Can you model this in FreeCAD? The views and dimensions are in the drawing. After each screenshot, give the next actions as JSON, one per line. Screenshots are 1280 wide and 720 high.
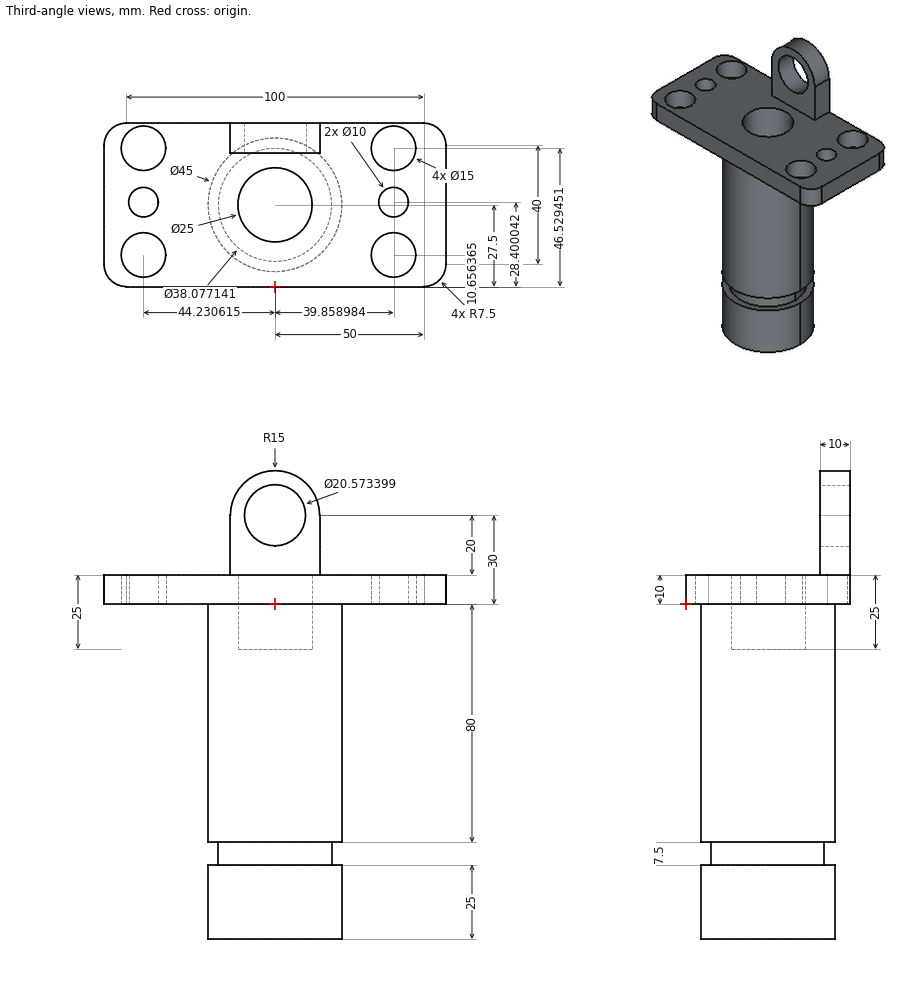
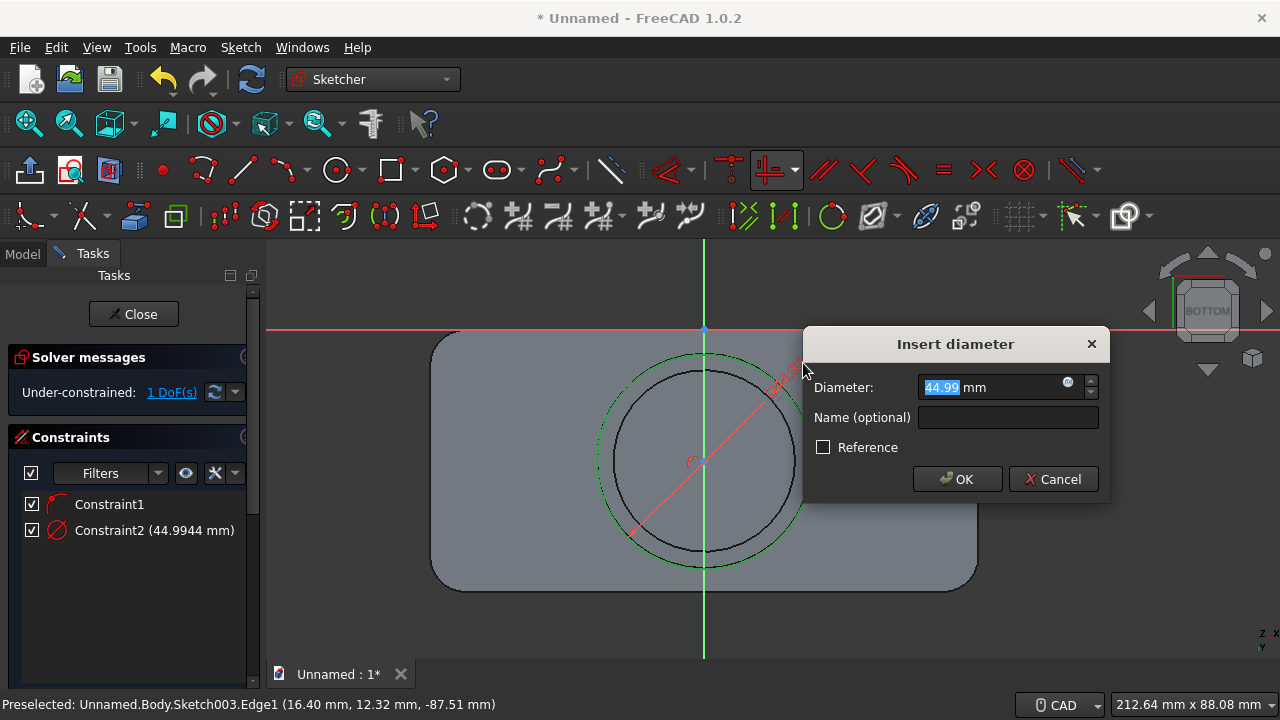
{"action": "type", "text": "45"}
{"action": "key", "text": "Return"}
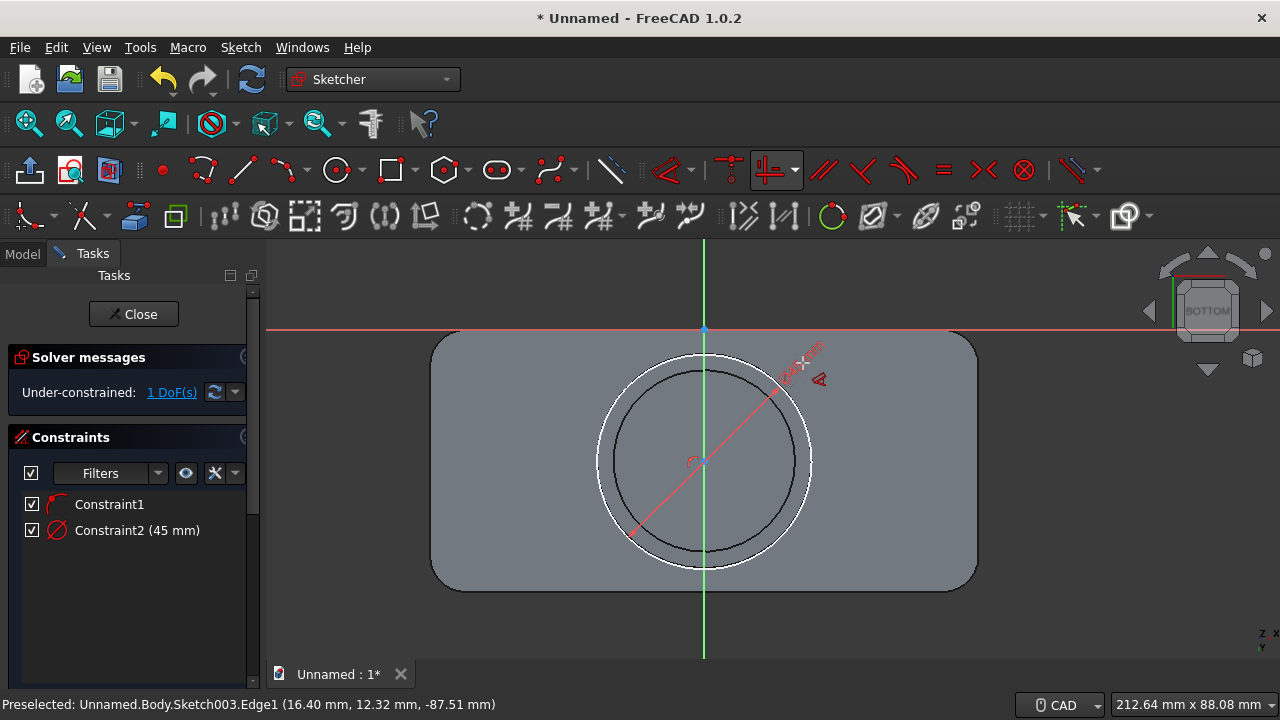
{"action": "left_click", "coordinate": [704, 462]}
{"action": "left_click", "coordinate": [738, 396]}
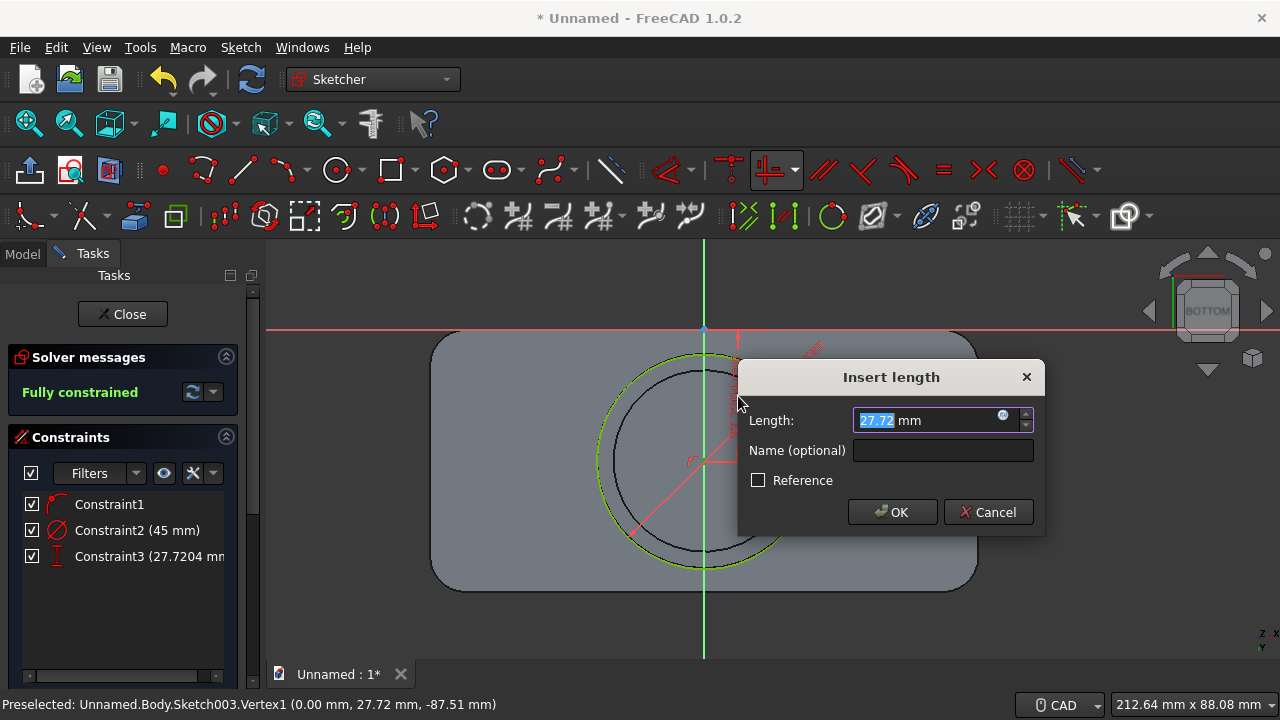
{"action": "type", "text": "27.5"}
{"action": "key", "text": "Return"}
{"action": "key", "text": "Escape"}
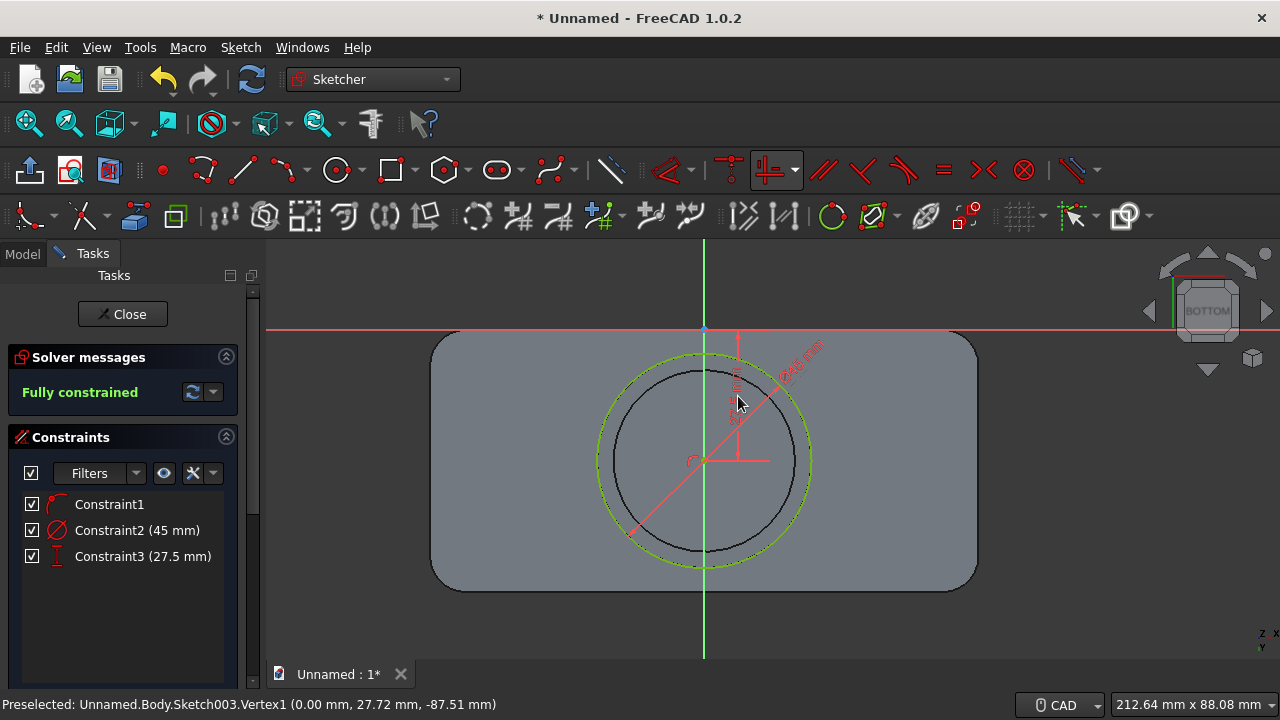
{"action": "left_click", "coordinate": [123, 314]}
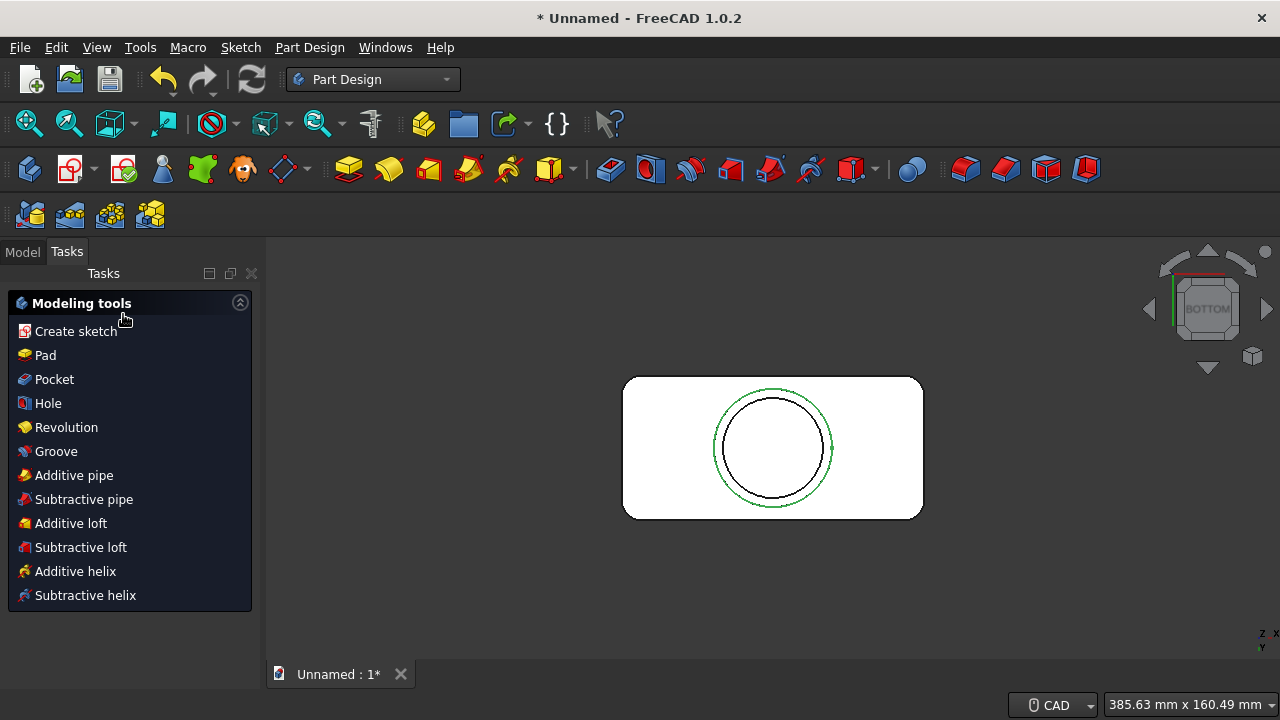
{"action": "left_click", "coordinate": [350, 170]}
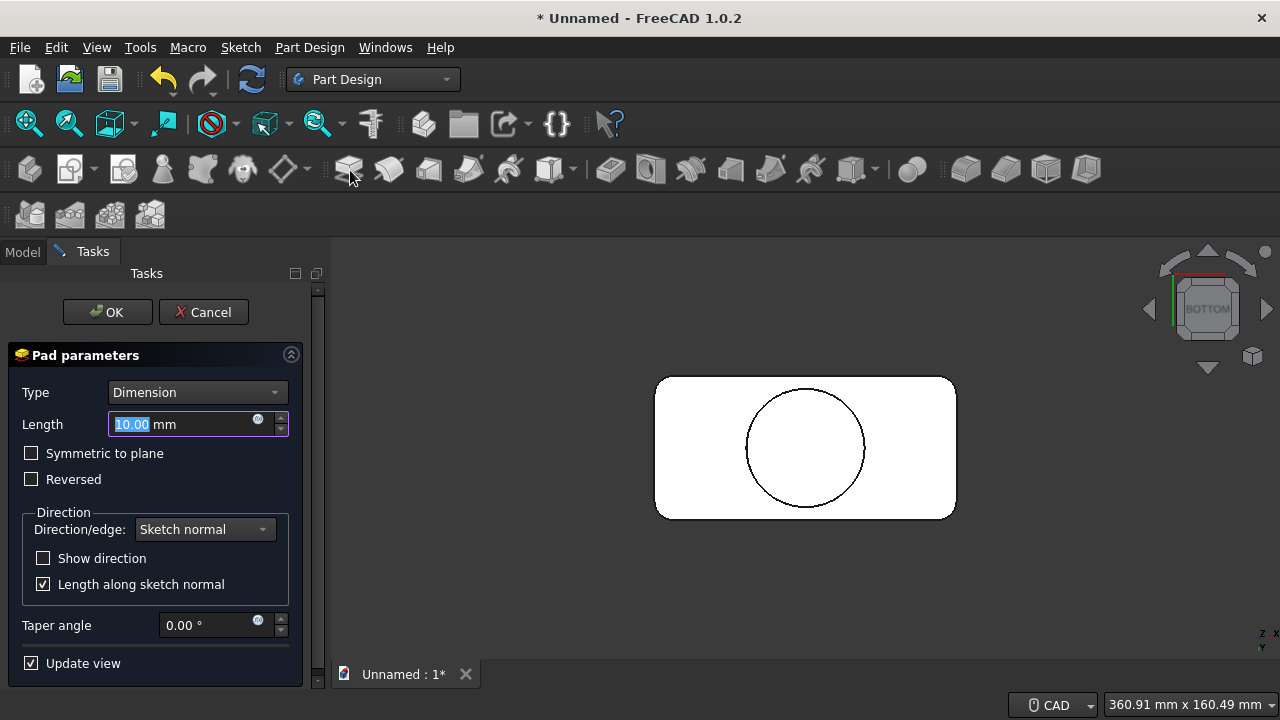
{"action": "type", "text": "25"}
{"action": "key", "text": "Tab"}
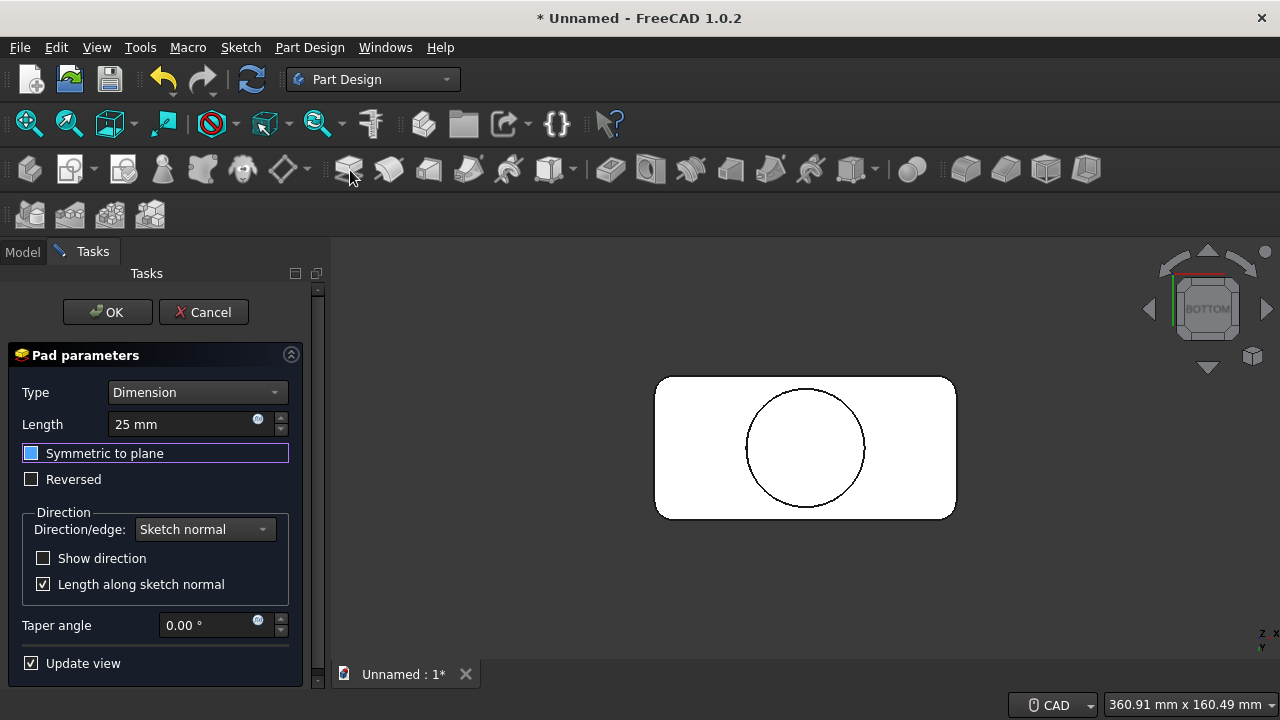
{"action": "left_click", "coordinate": [108, 312]}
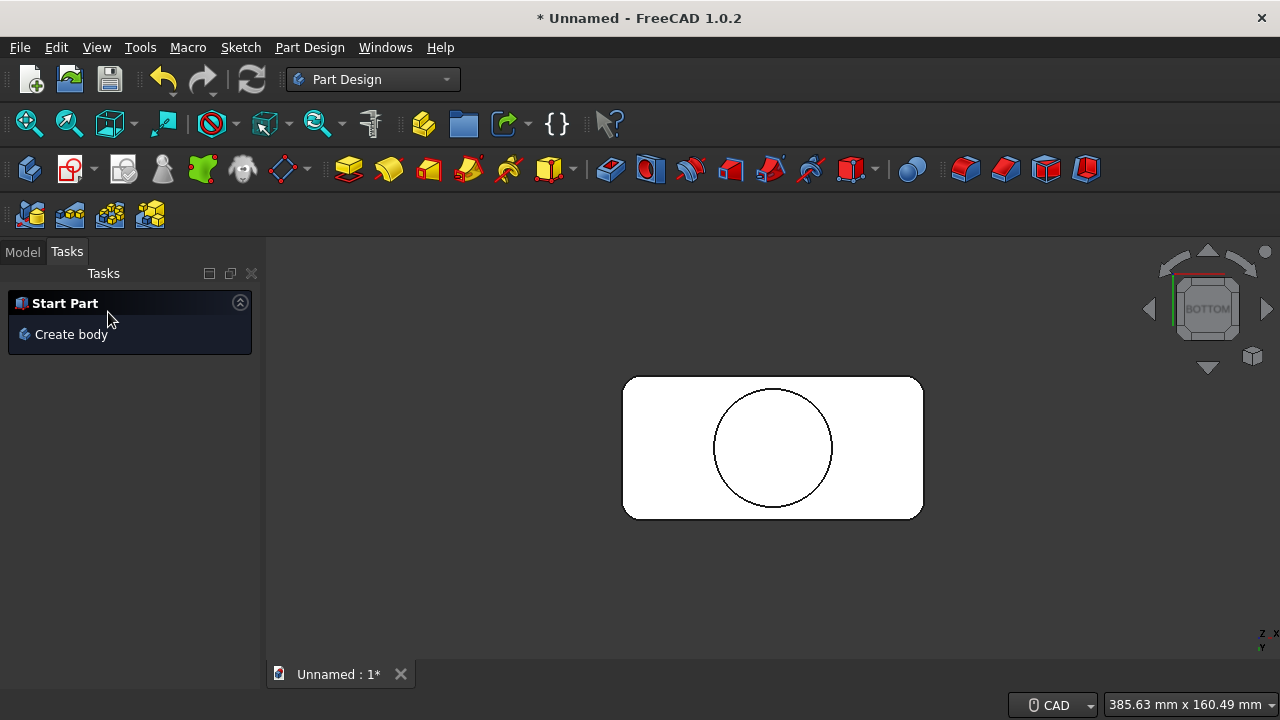
{"action": "key", "text": "v f"}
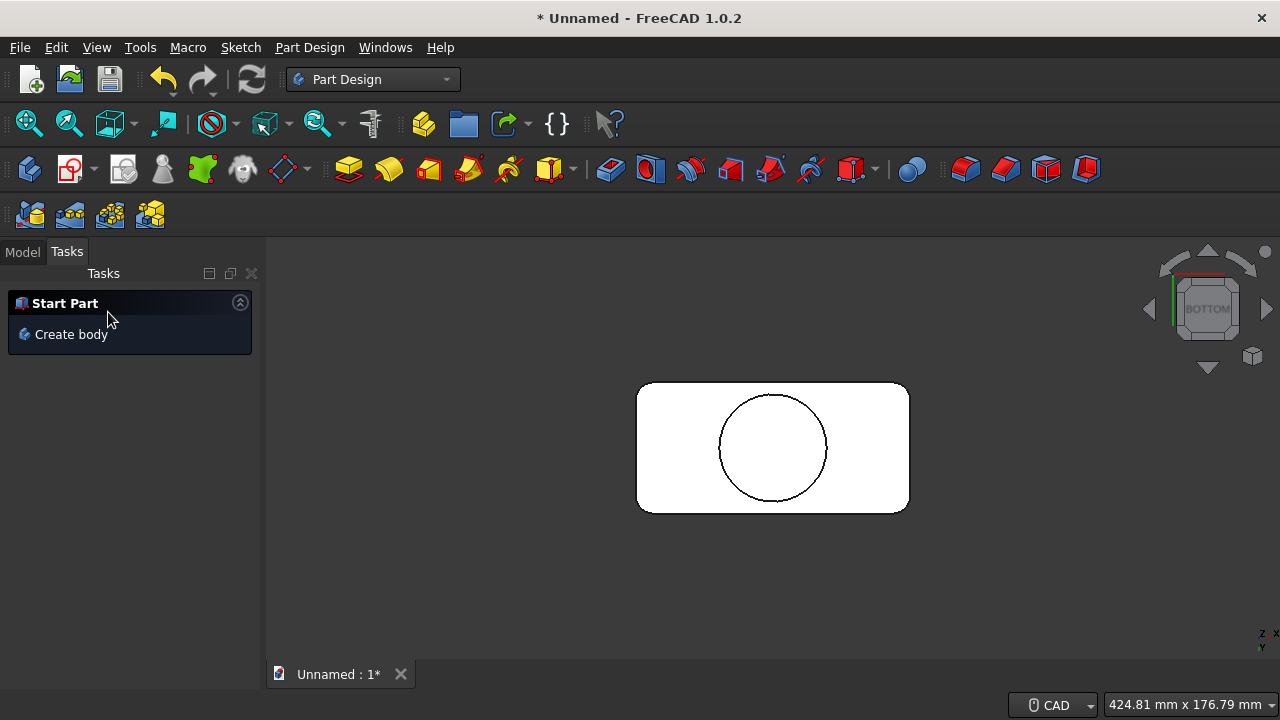
{"action": "key", "text": "0"}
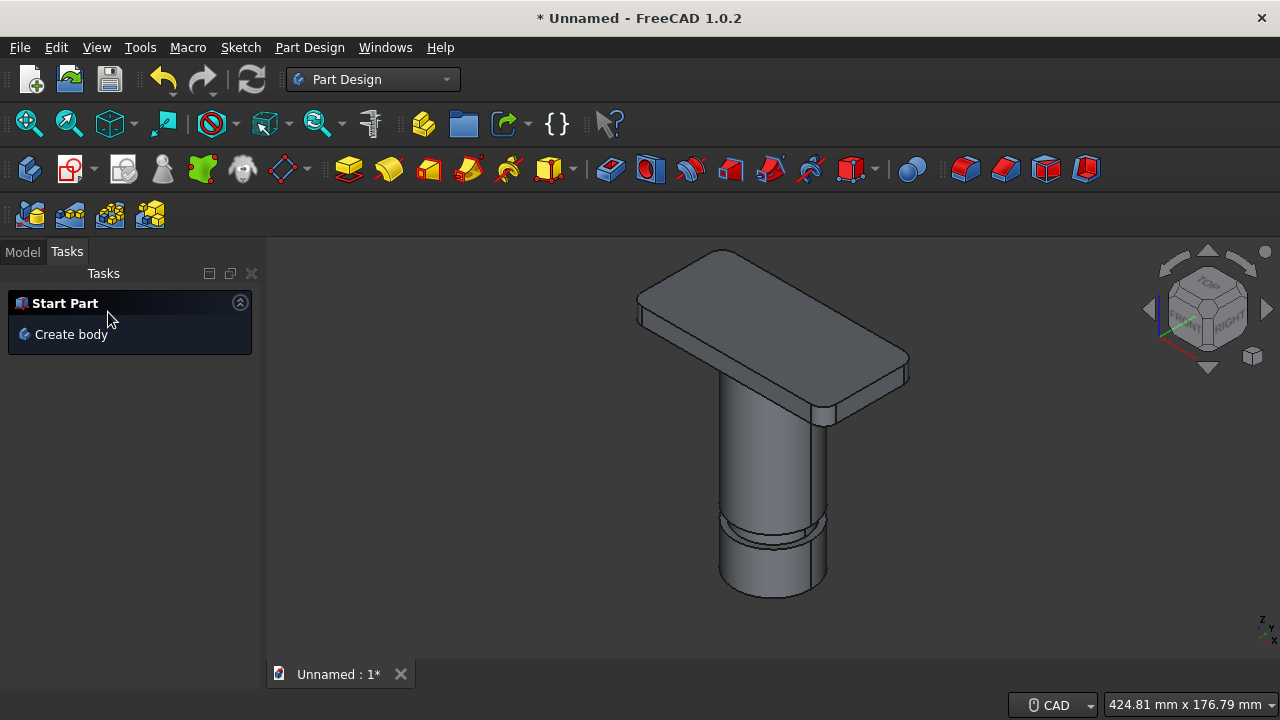
{"action": "left_click", "coordinate": [801, 344]}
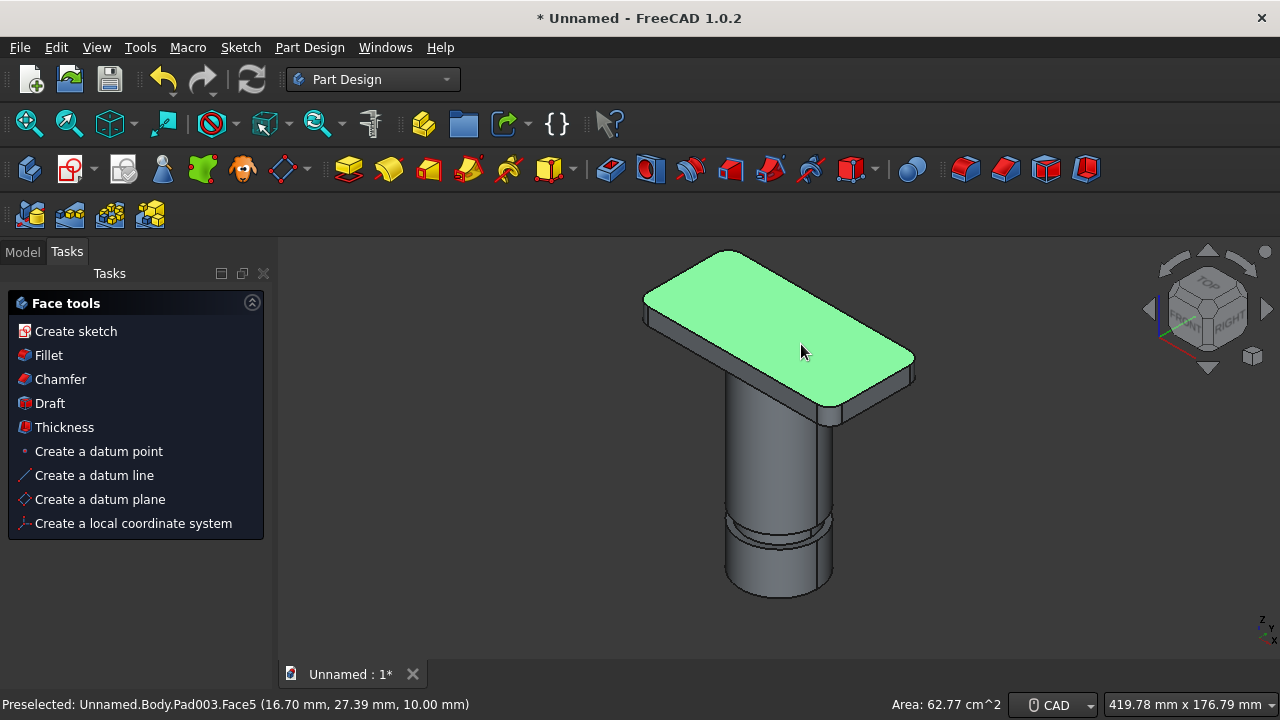
{"action": "left_click", "coordinate": [70, 170]}